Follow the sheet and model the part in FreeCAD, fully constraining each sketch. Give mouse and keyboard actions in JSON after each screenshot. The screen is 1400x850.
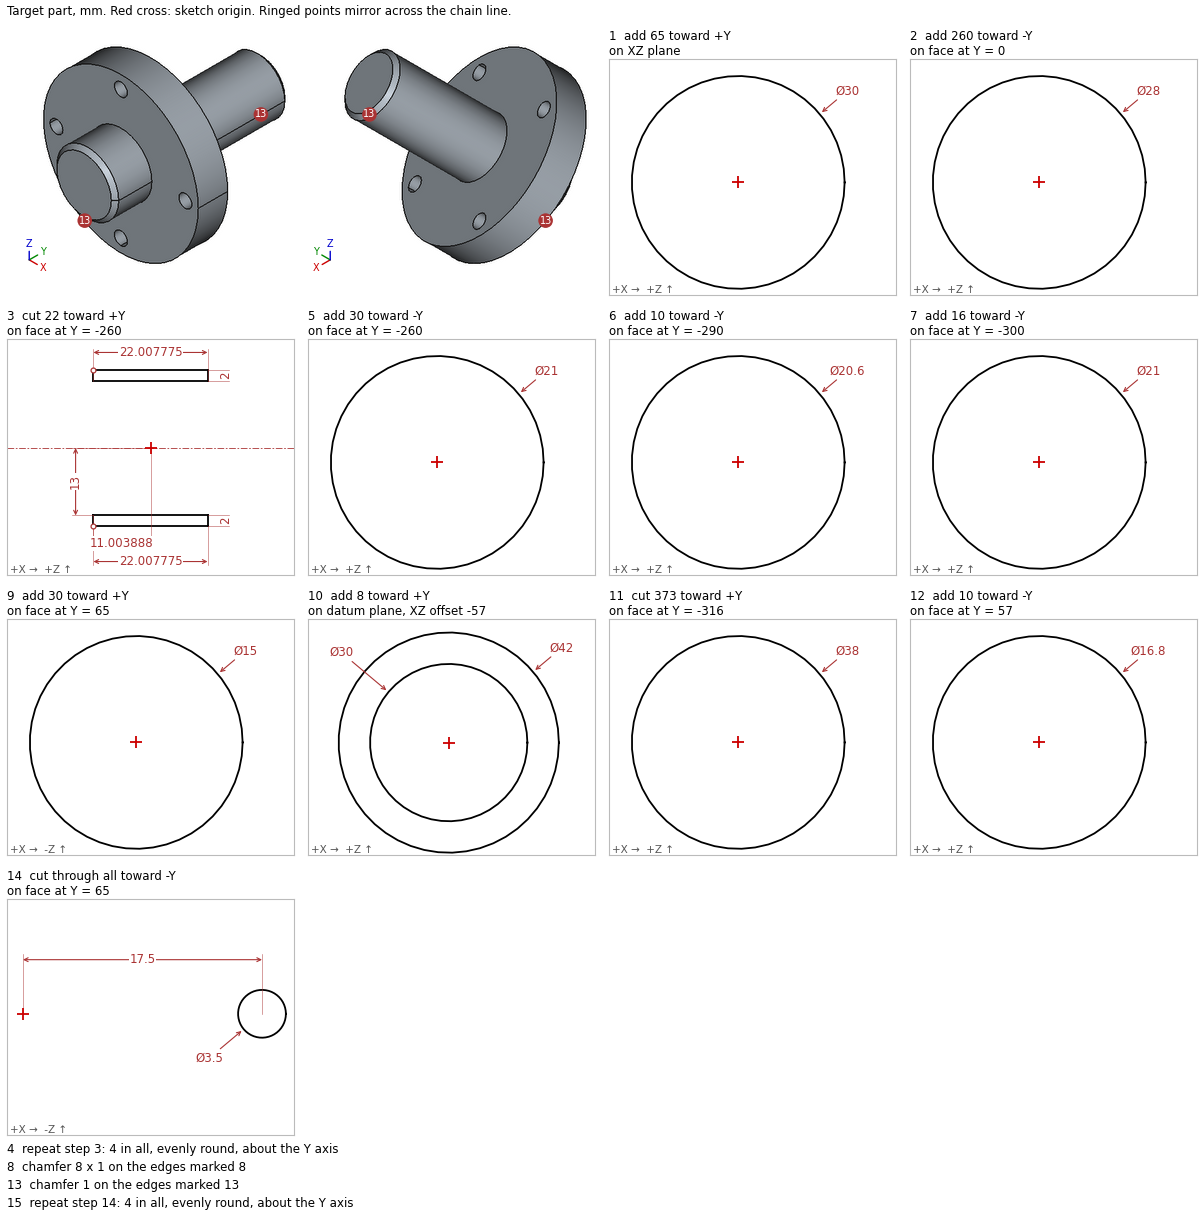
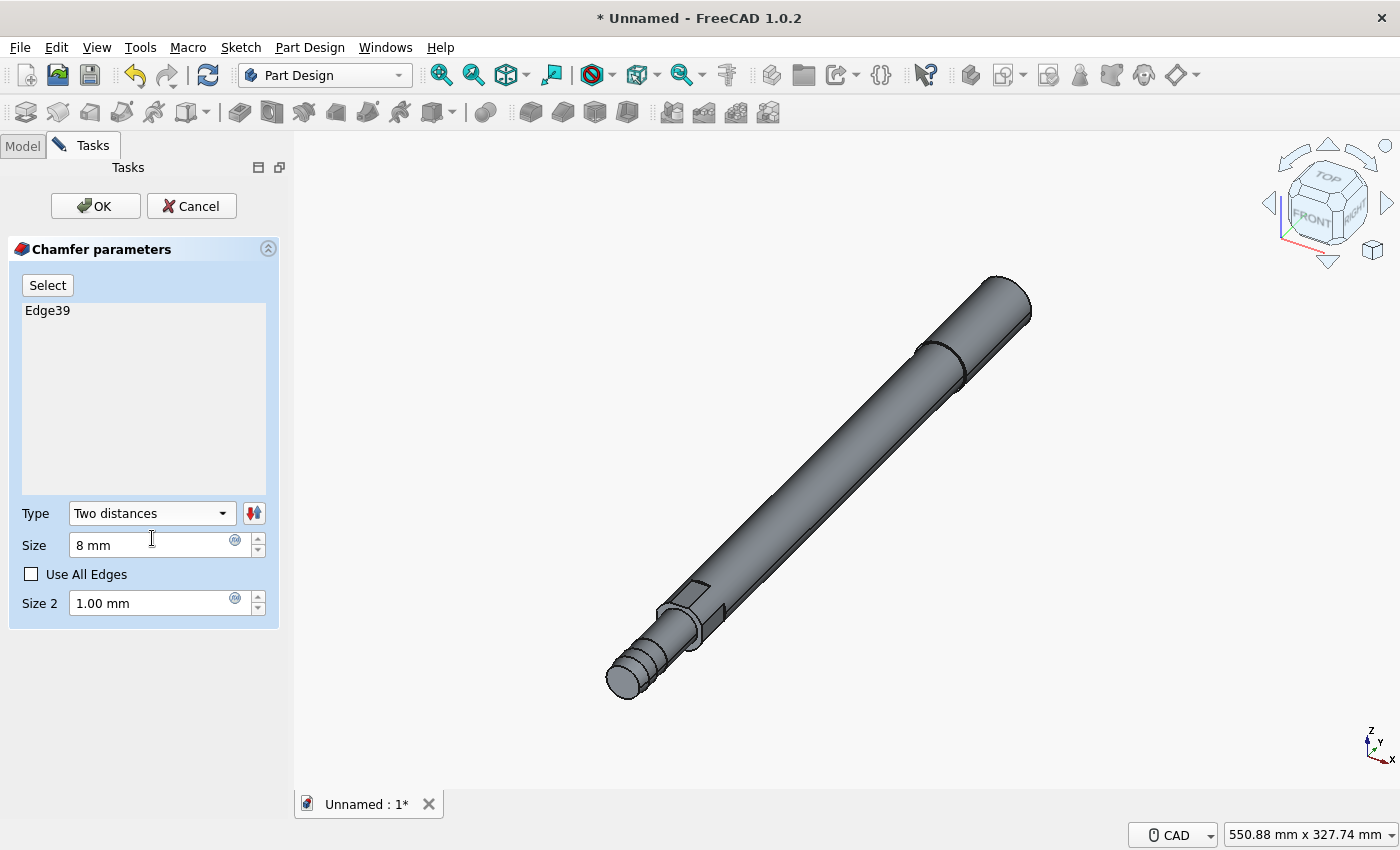
{"action": "triple_click", "coordinate": [160, 603]}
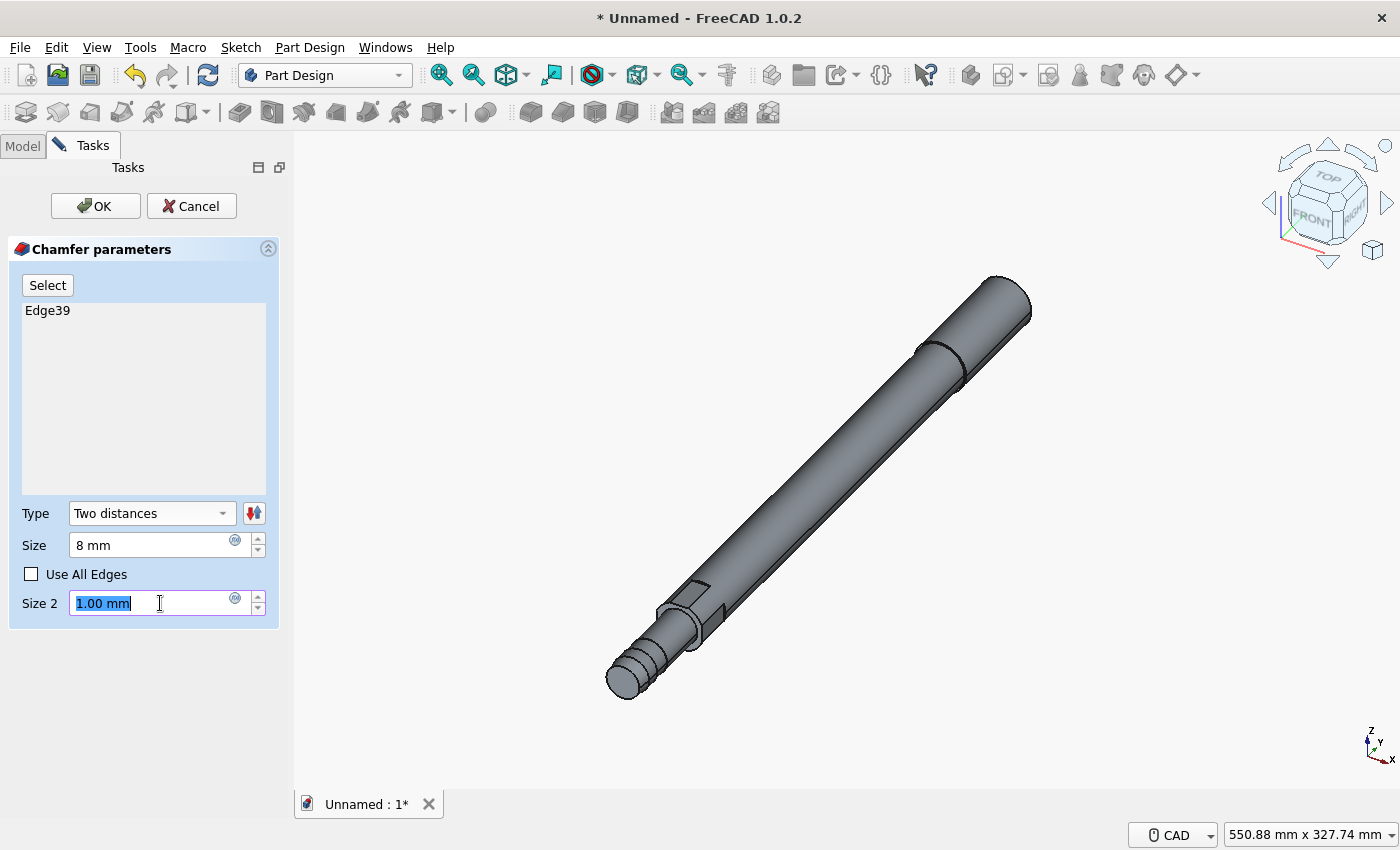
{"action": "type", "text": "1"}
{"action": "key", "text": "Tab"}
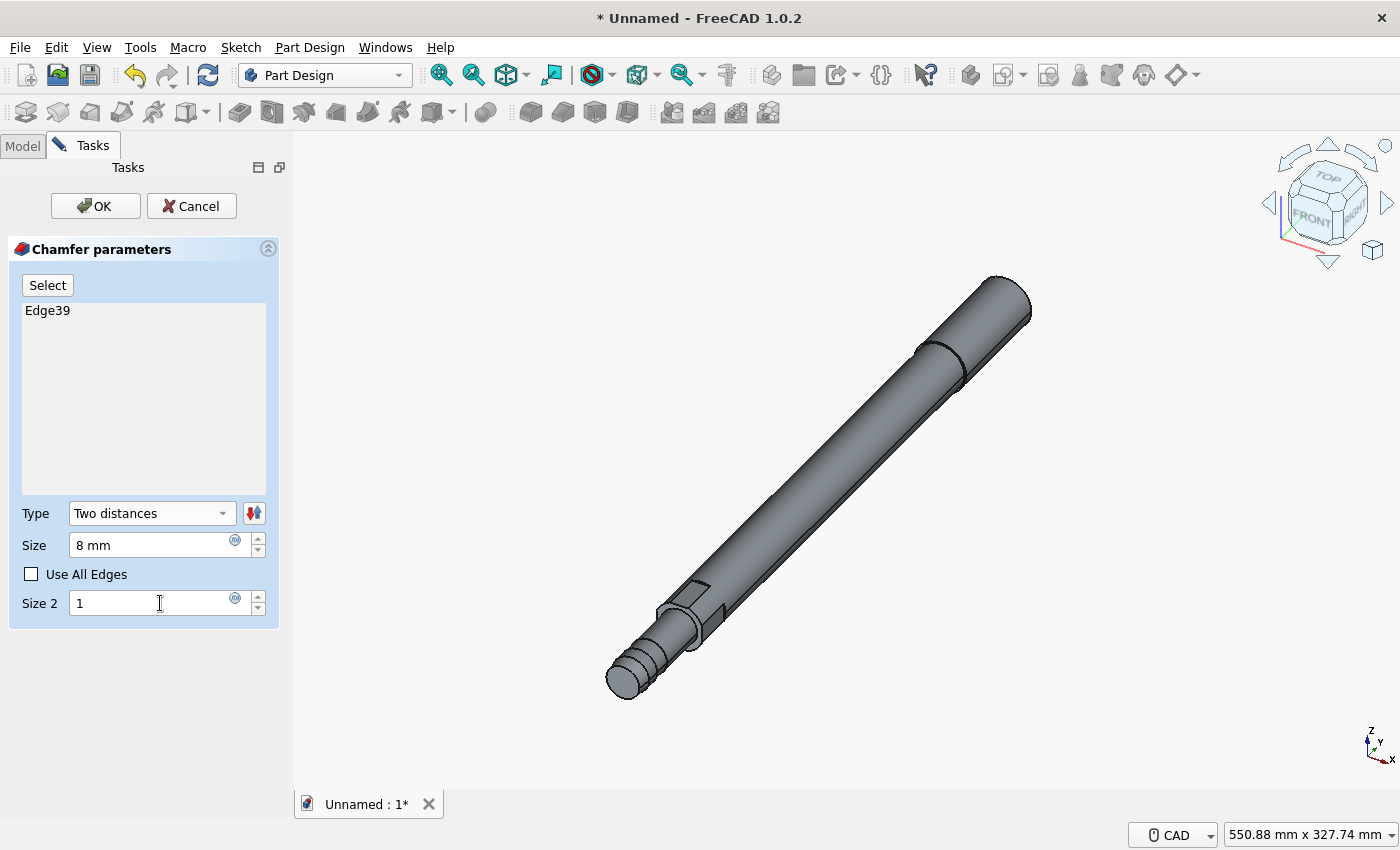
{"action": "left_click", "coordinate": [96, 206]}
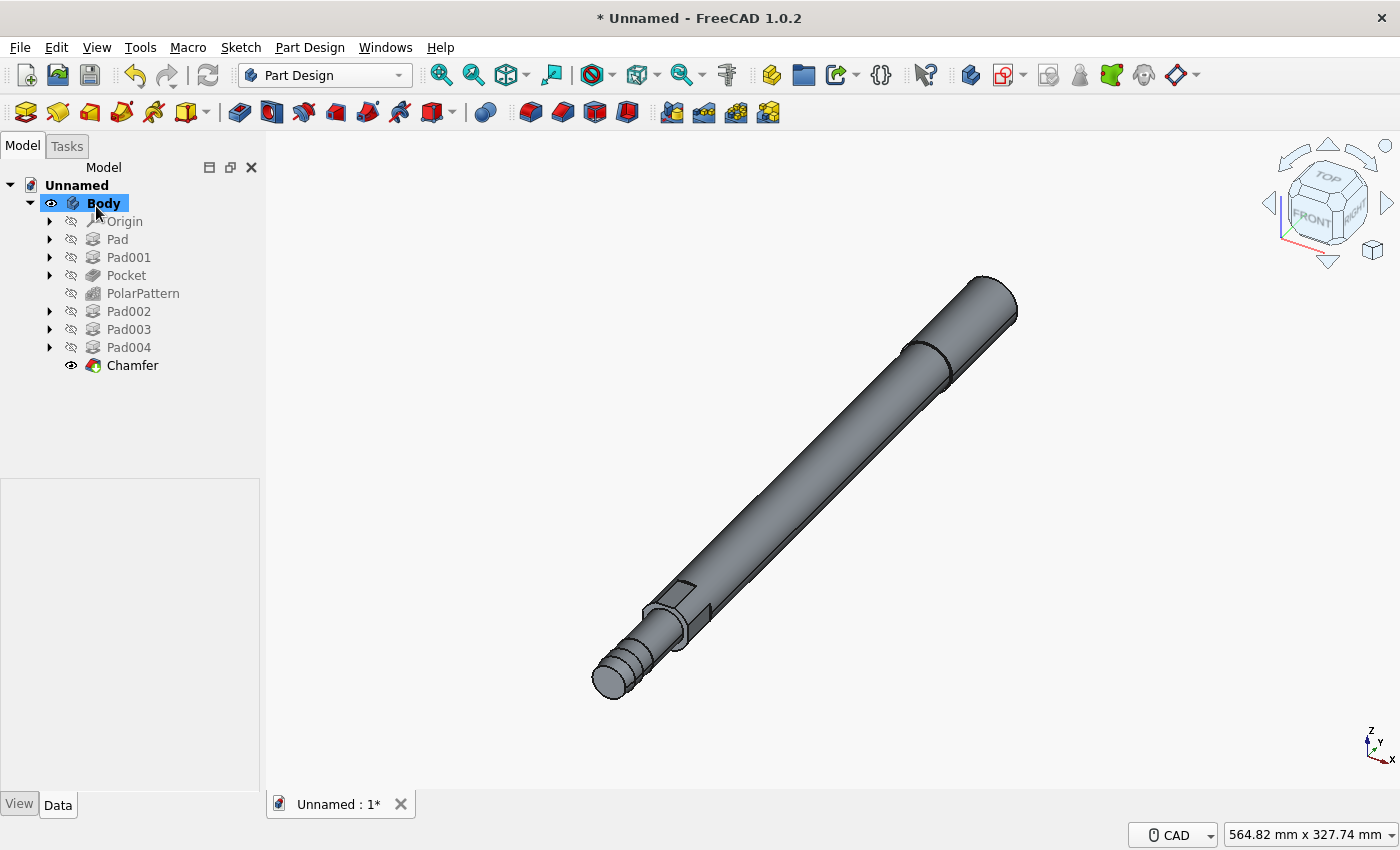
{"action": "key", "text": "4"}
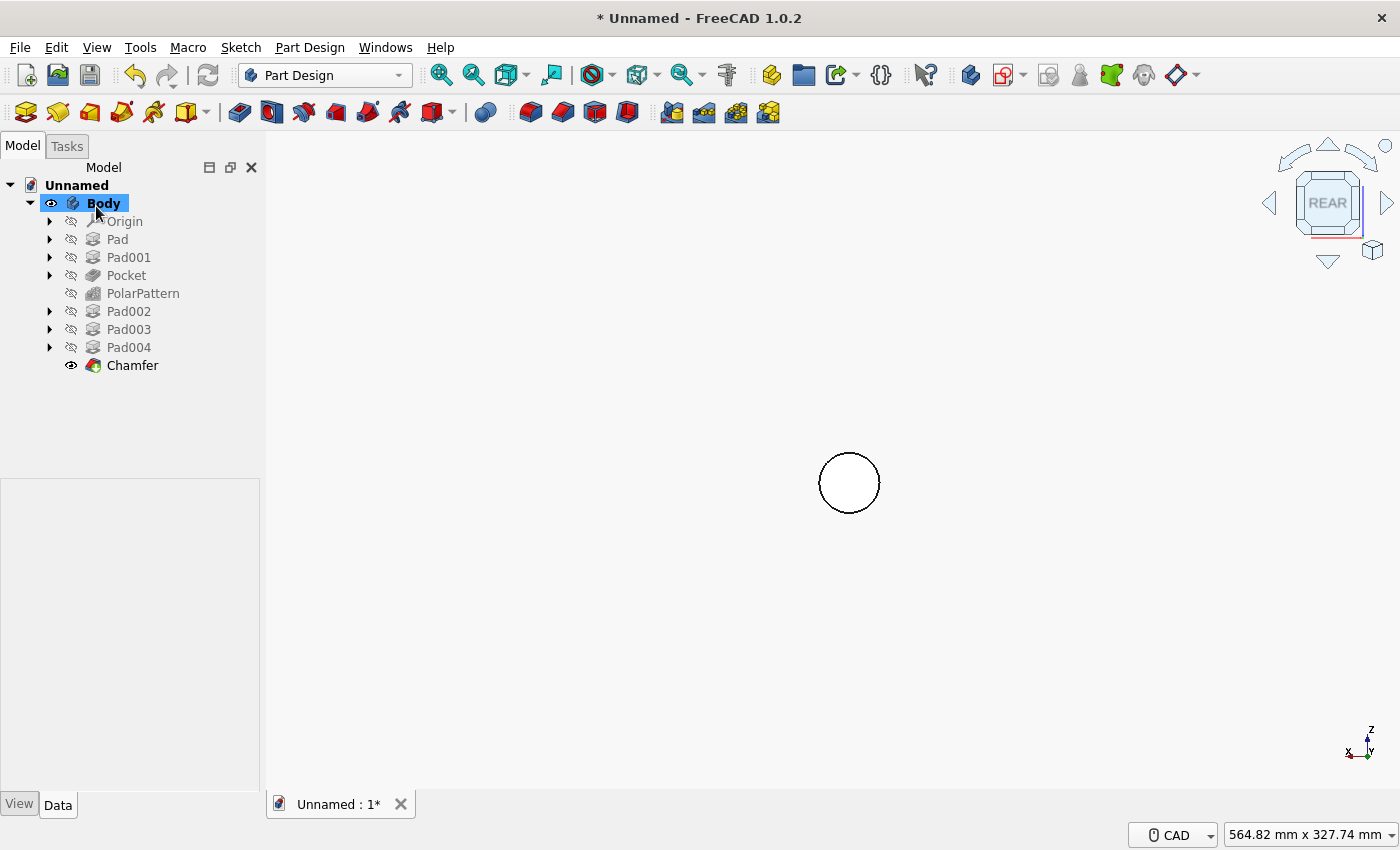
{"action": "key", "text": "v f"}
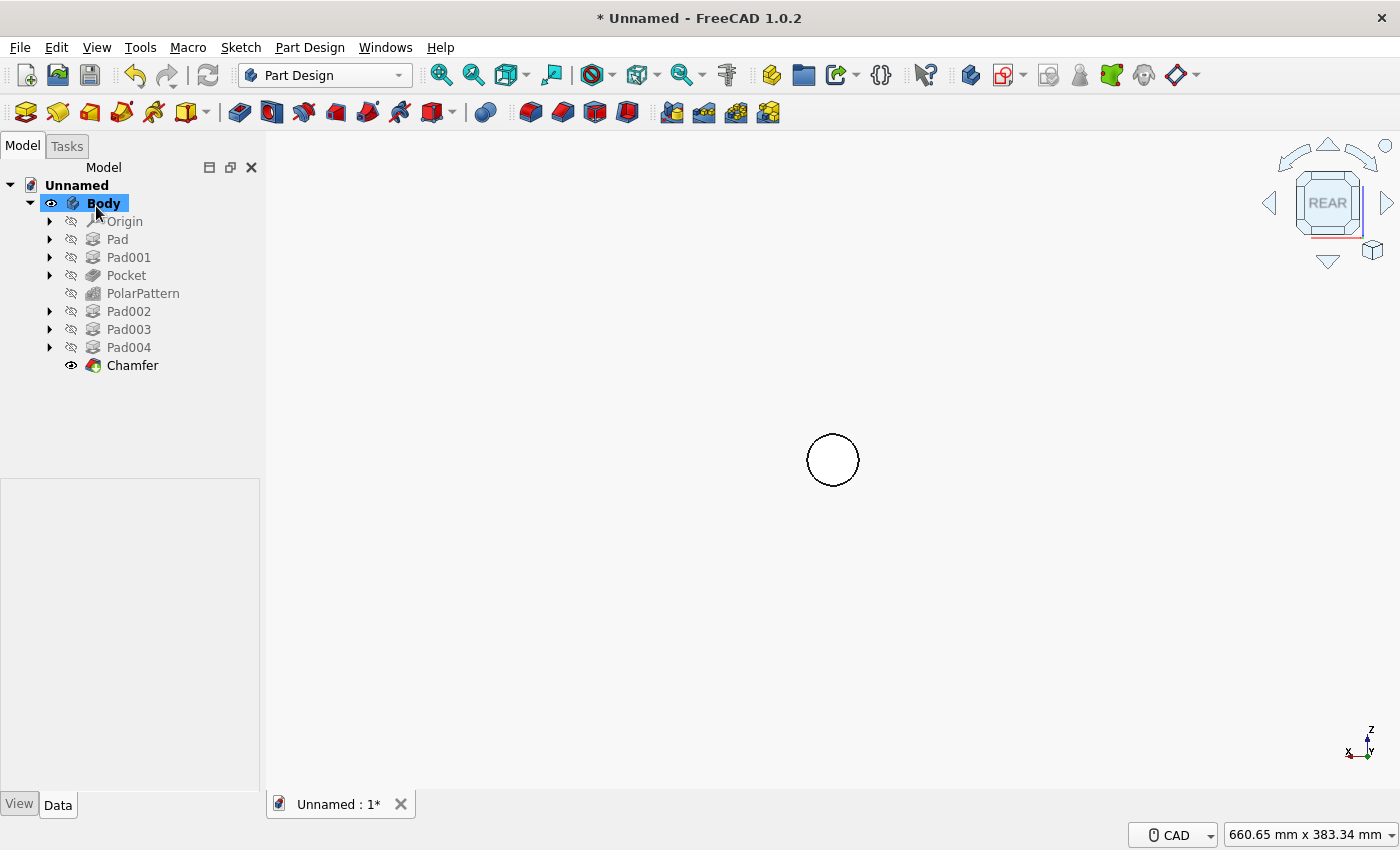
{"action": "left_click", "coordinate": [833, 459]}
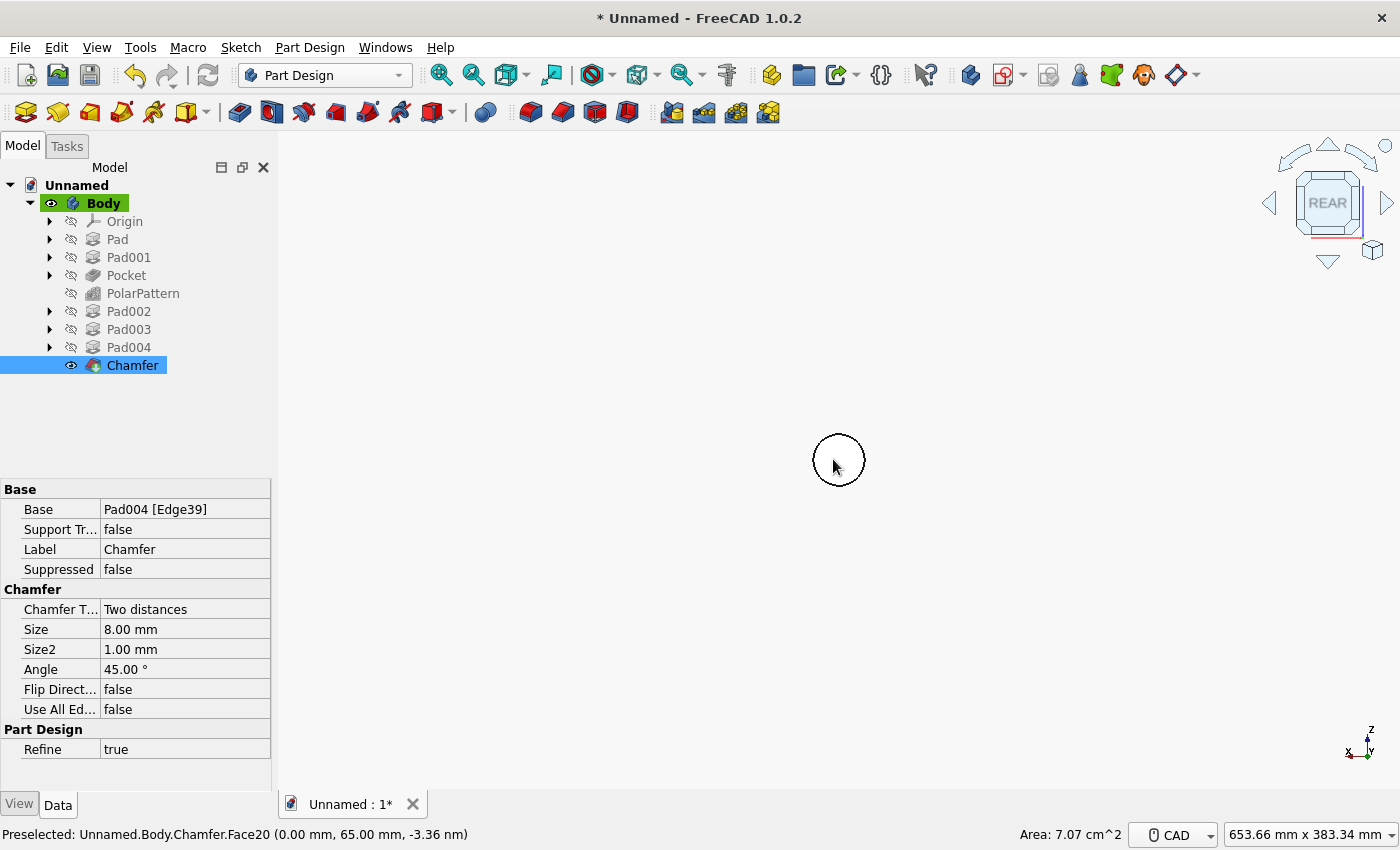
{"action": "left_click", "coordinate": [1004, 76]}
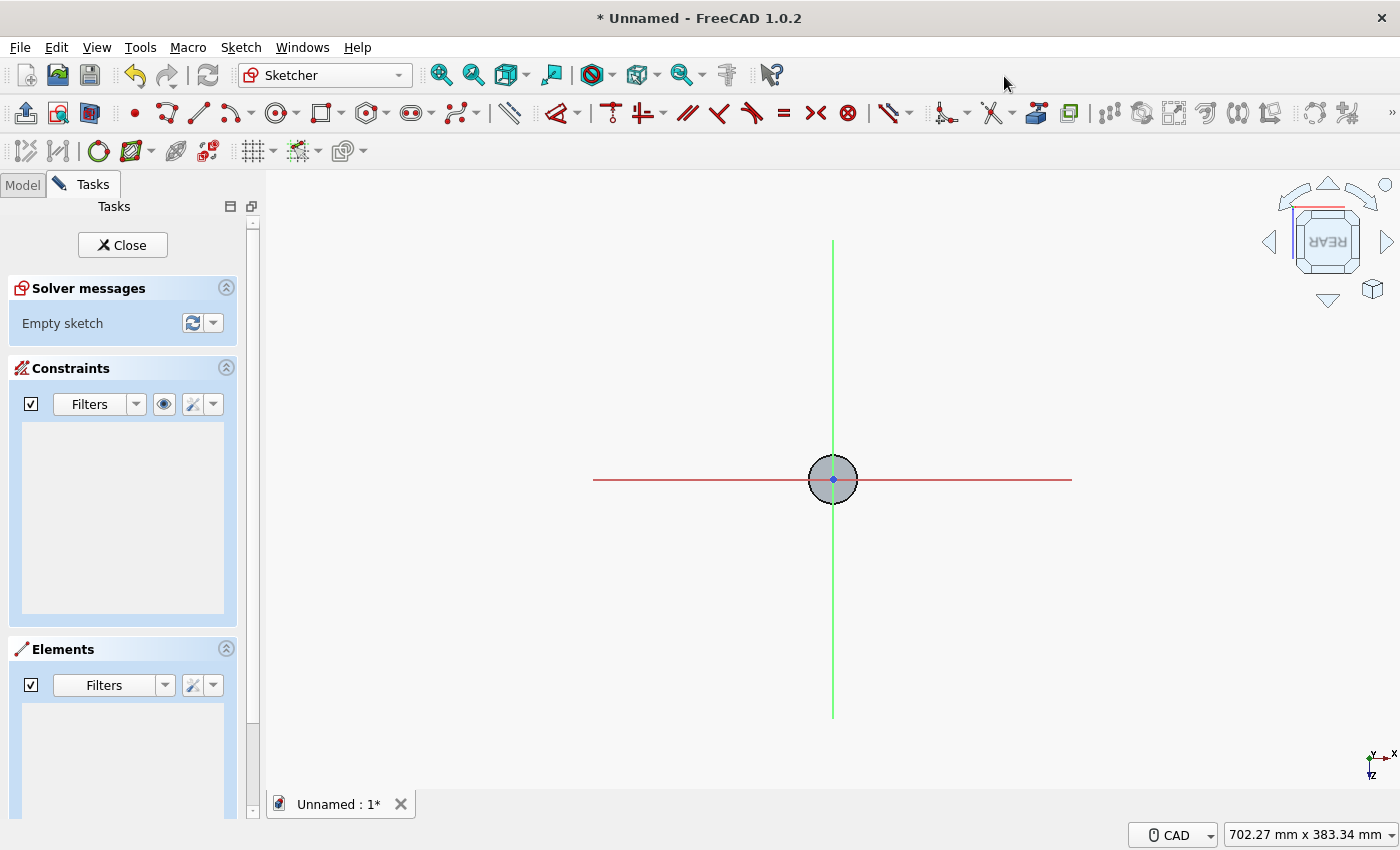
{"action": "scroll", "coordinate": [837, 480], "scroll_direction": "up", "scroll_amount": 14}